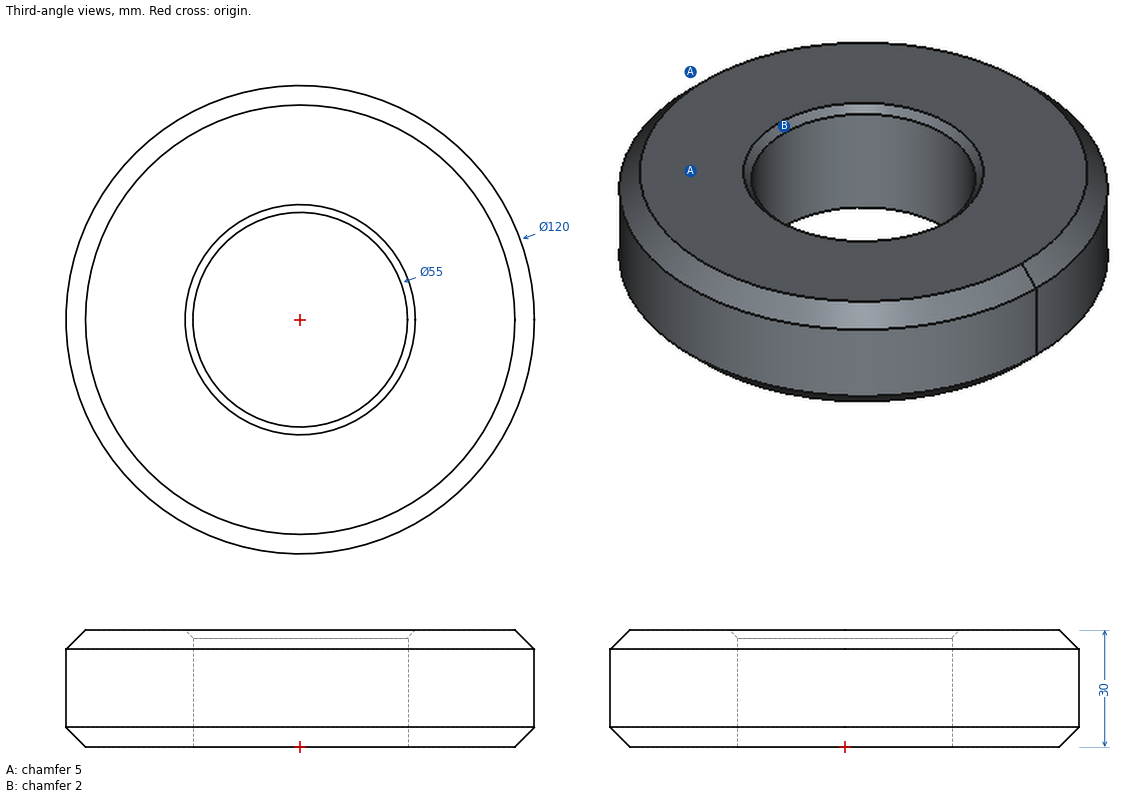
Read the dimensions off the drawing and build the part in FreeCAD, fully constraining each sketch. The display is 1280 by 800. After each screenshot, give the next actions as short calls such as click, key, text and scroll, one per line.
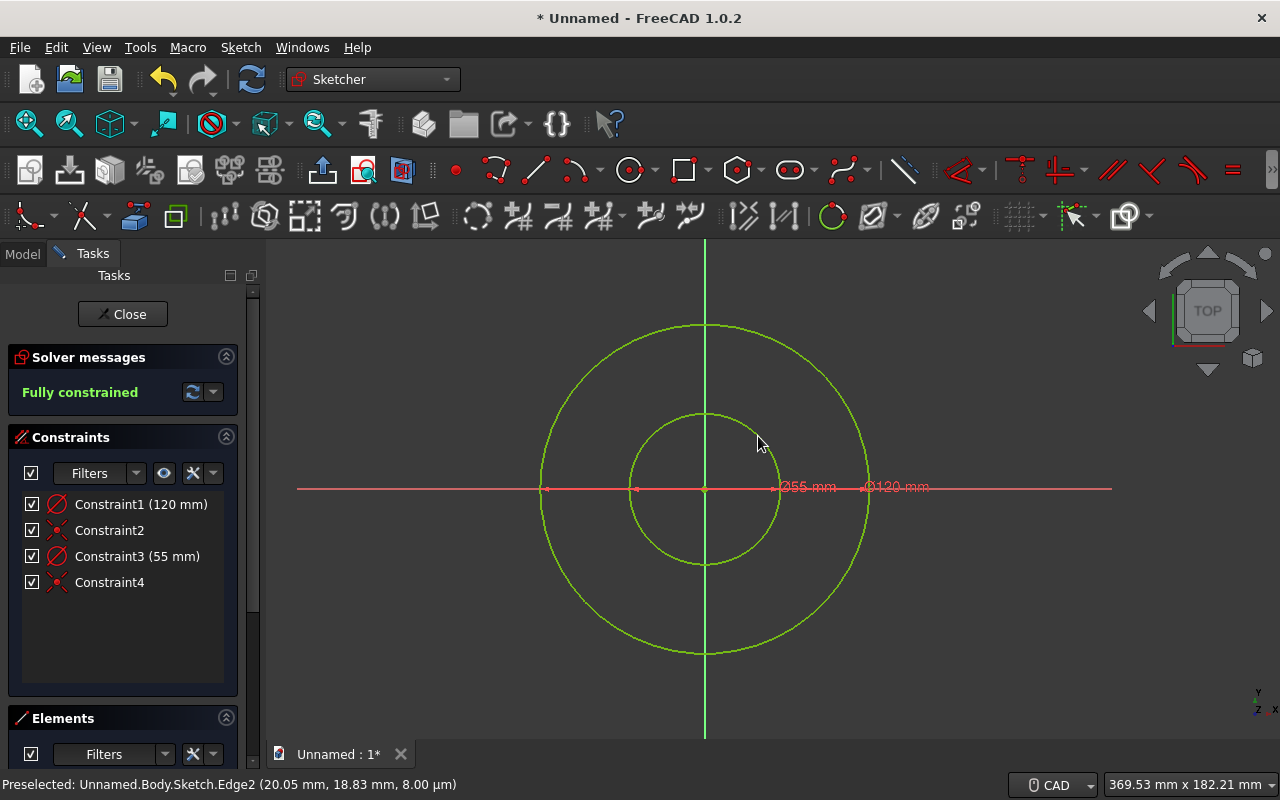
click(123, 314)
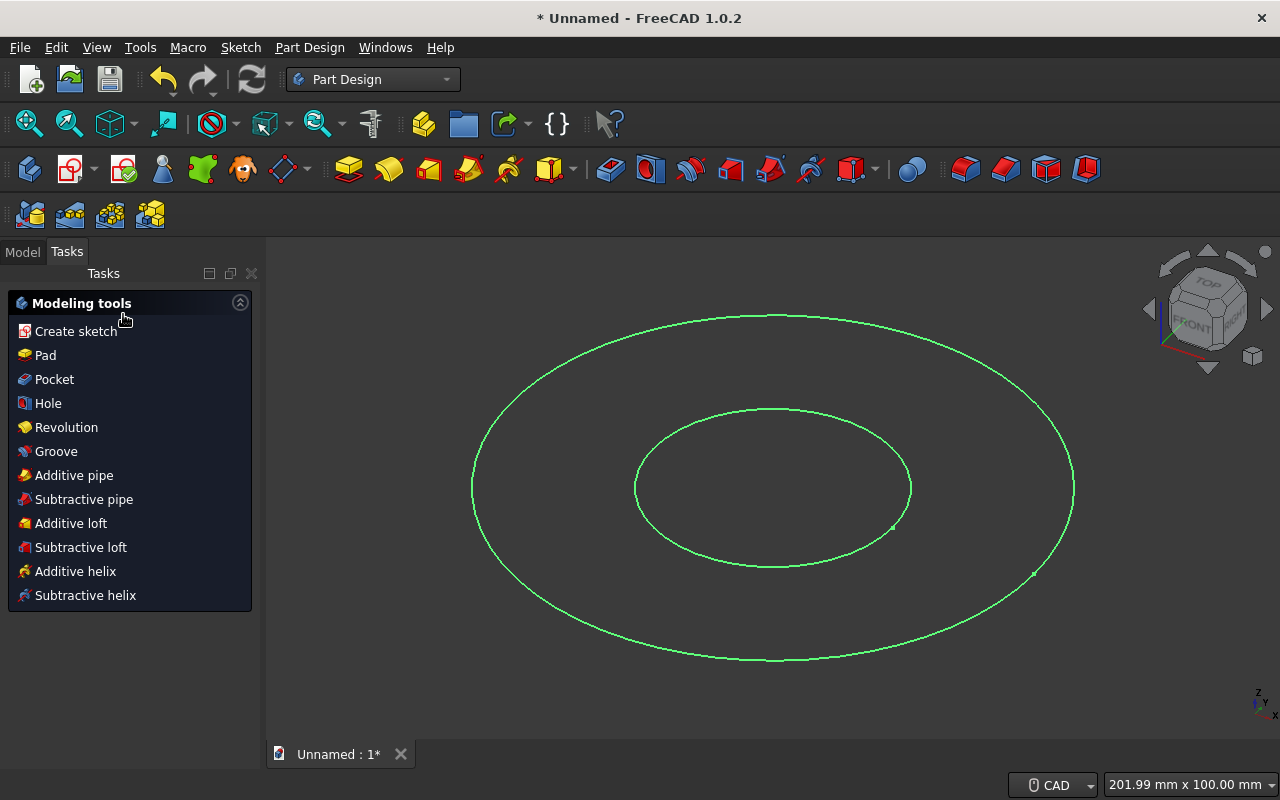
click(350, 170)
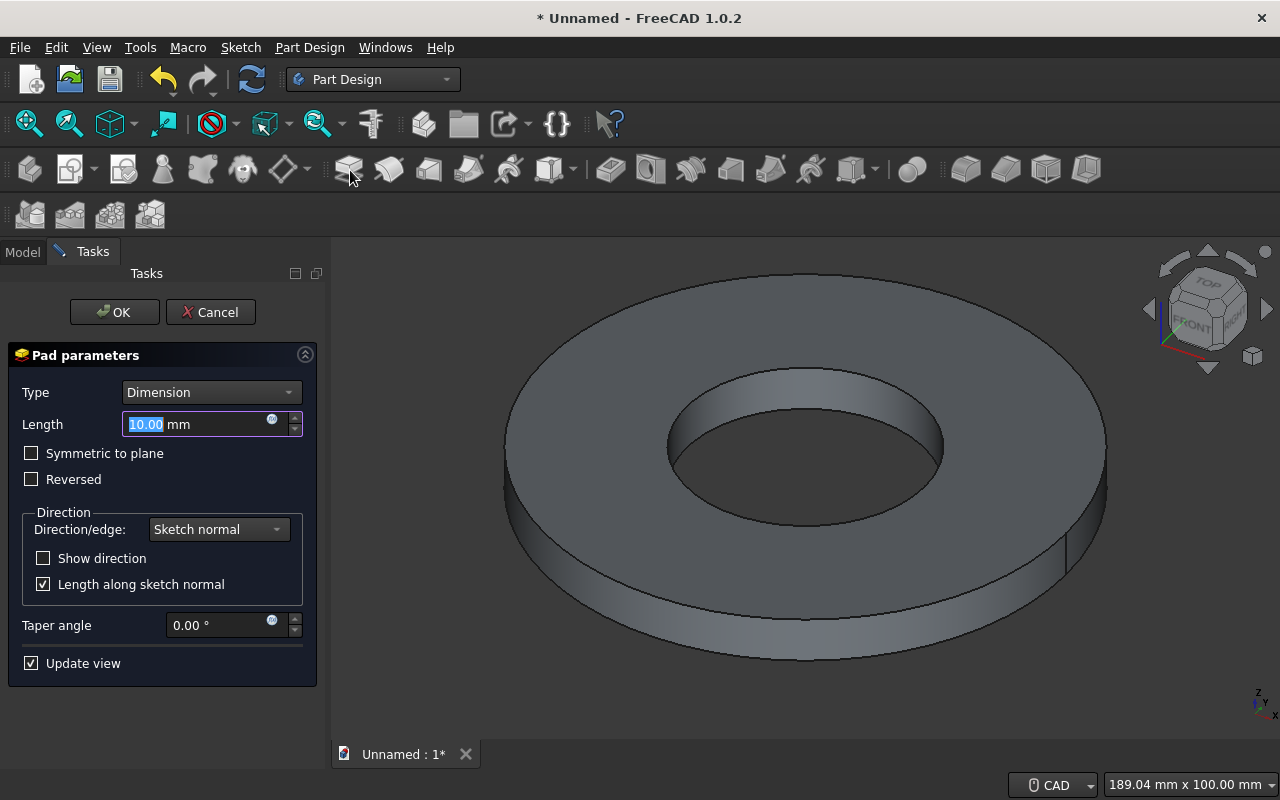
text(30)
key(Tab)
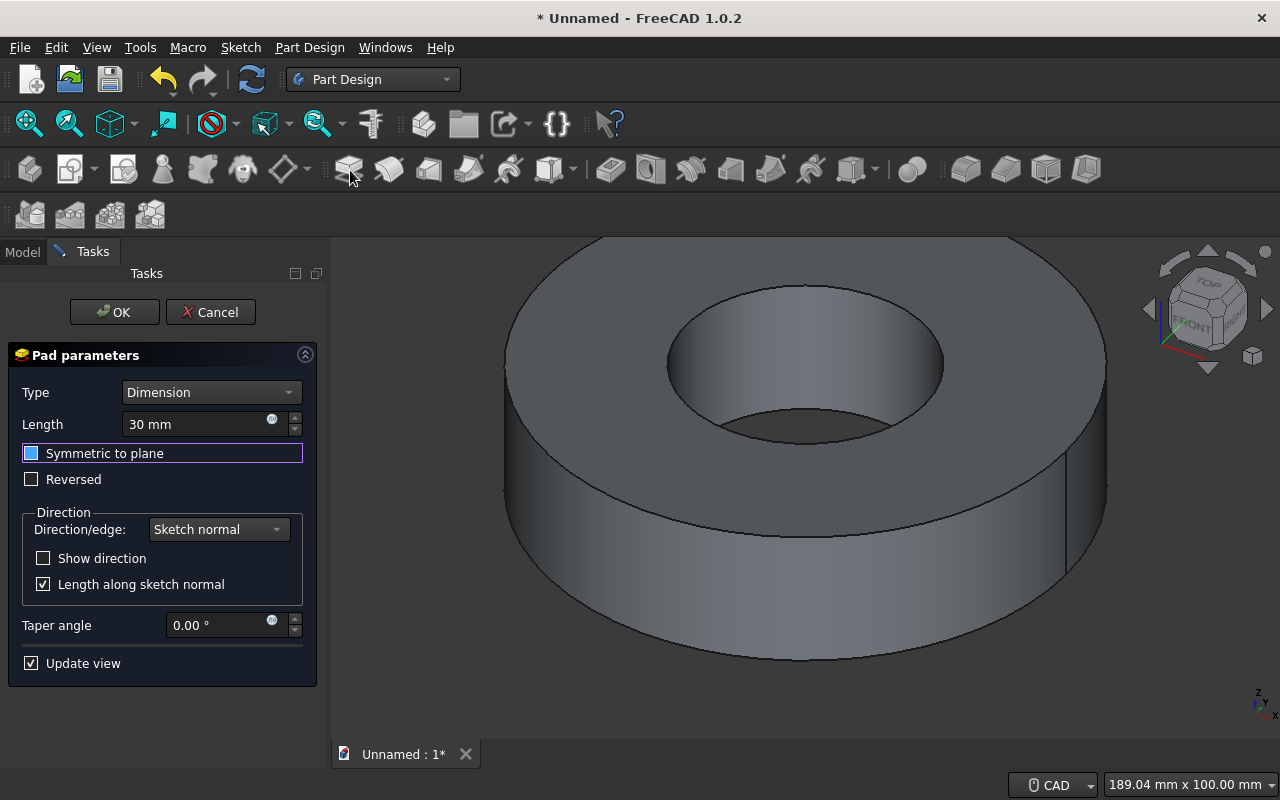
click(115, 312)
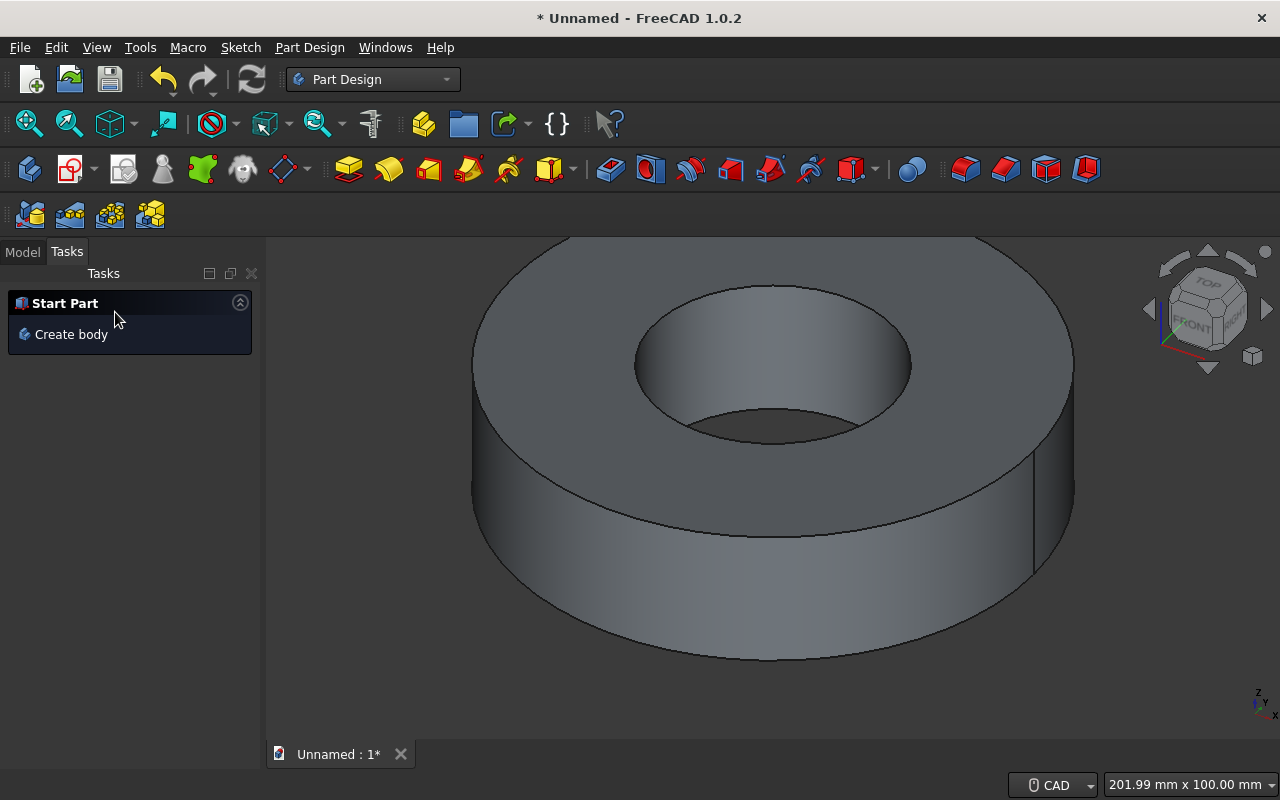
click(30, 124)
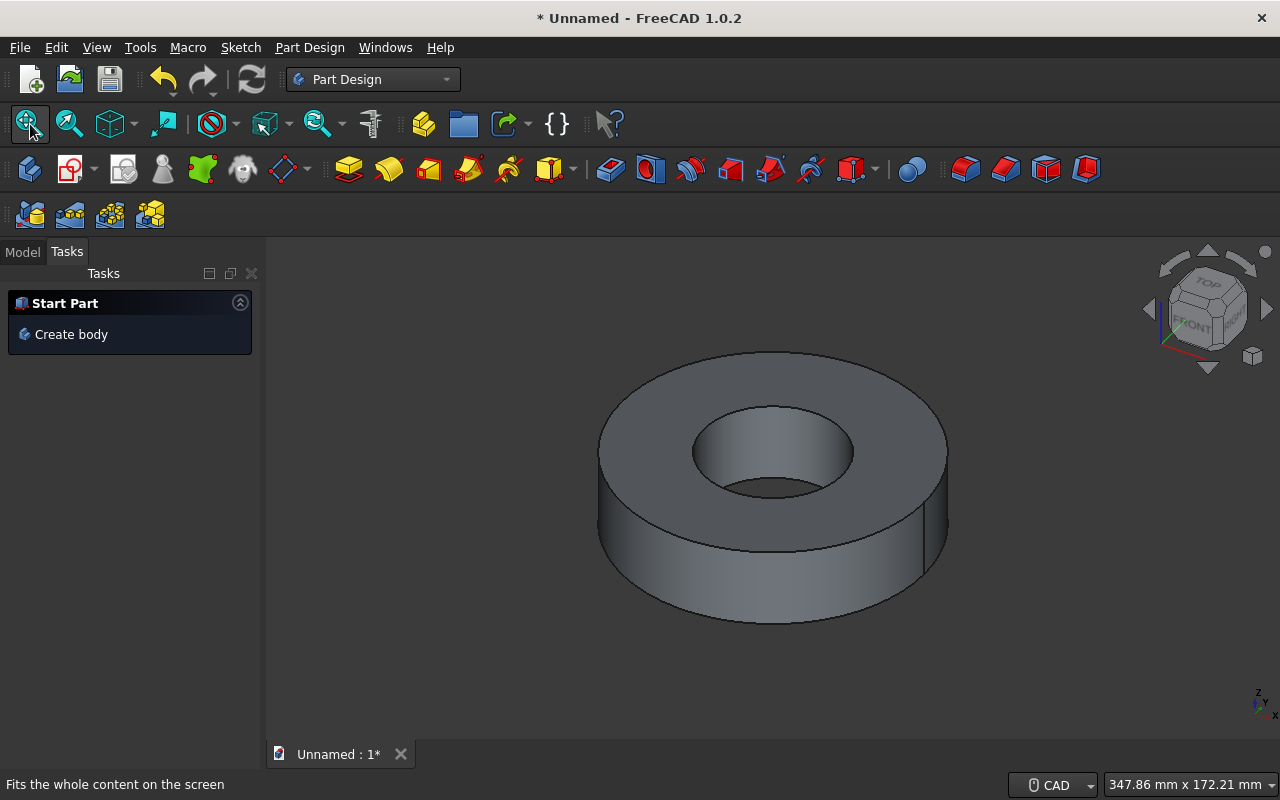
click(599, 462)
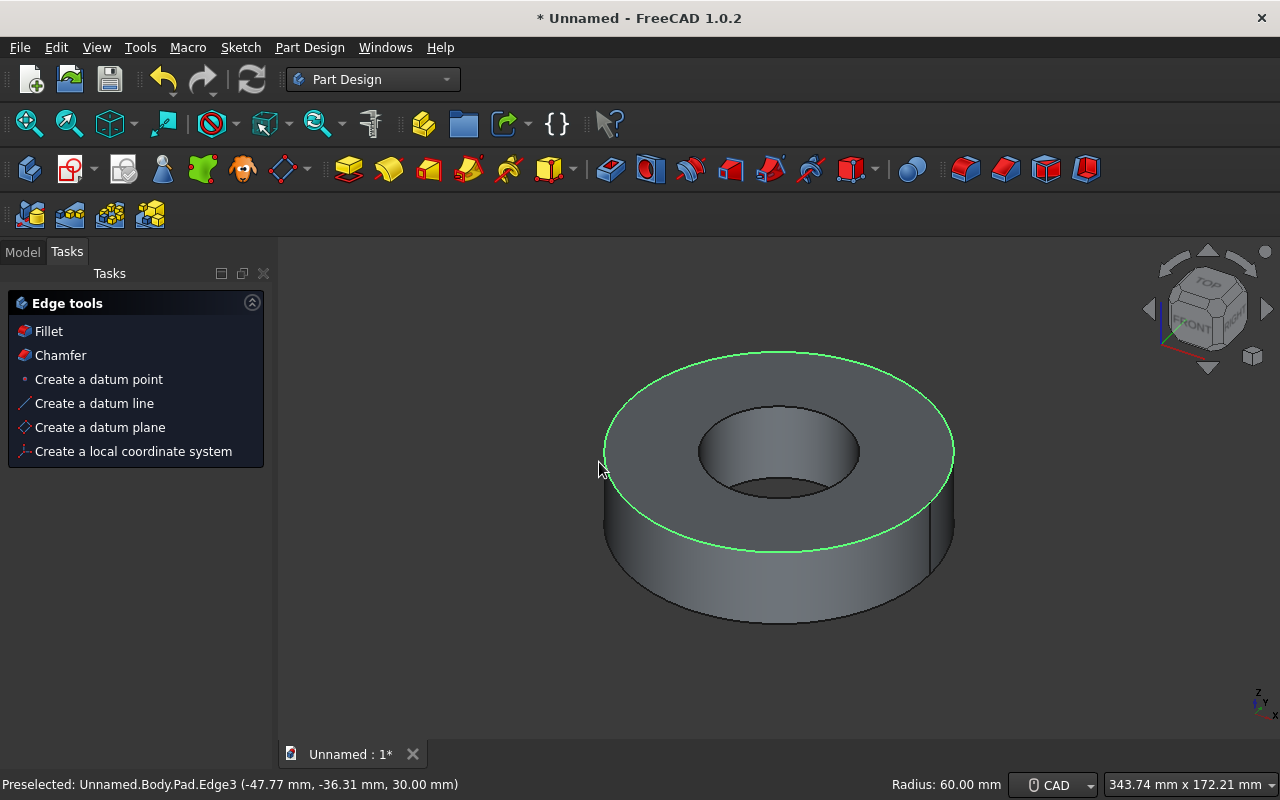
key(0)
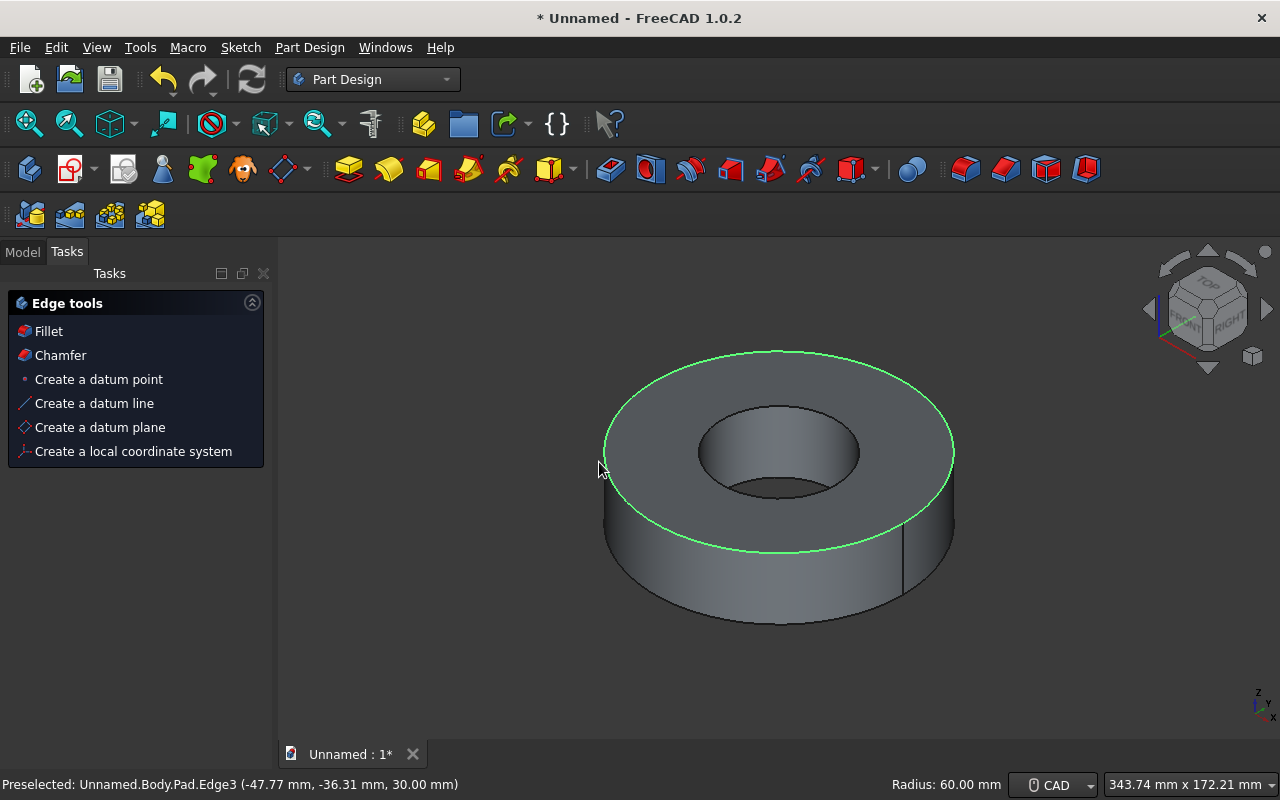
key(2)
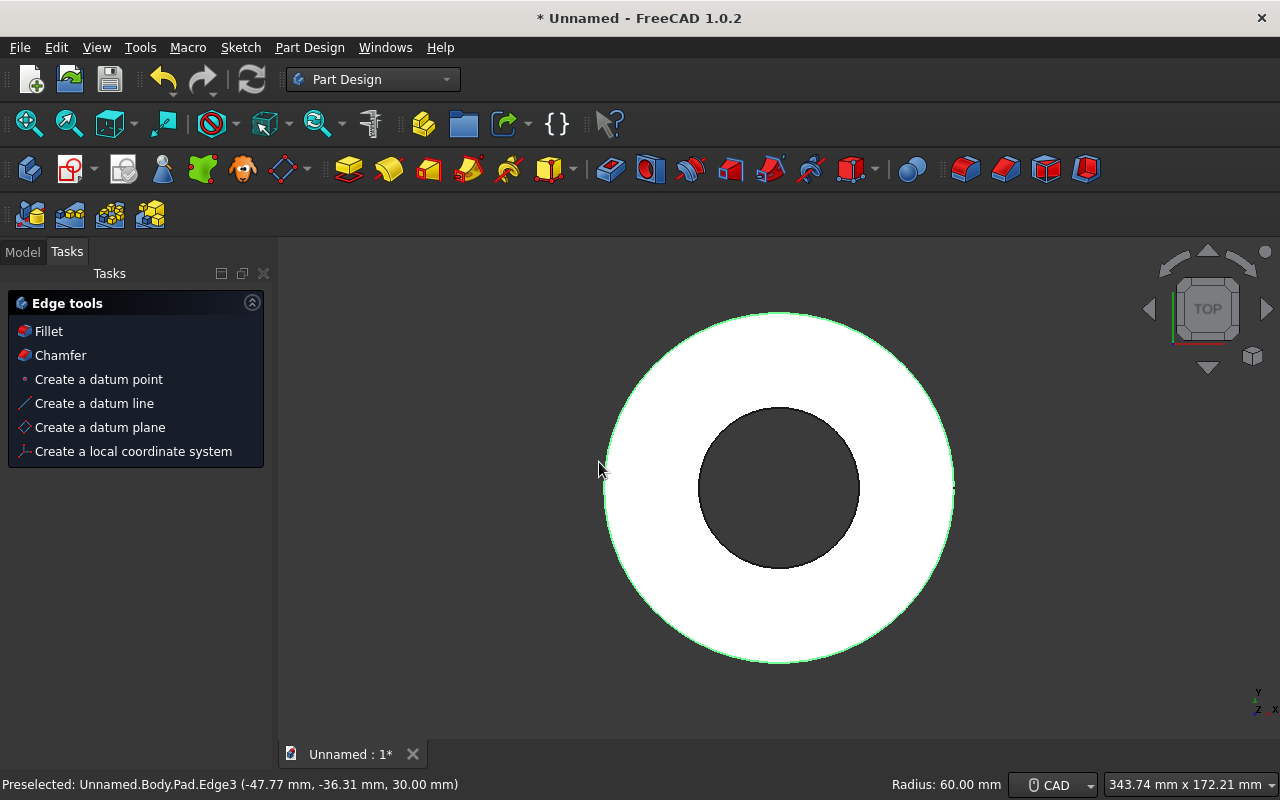
key(1)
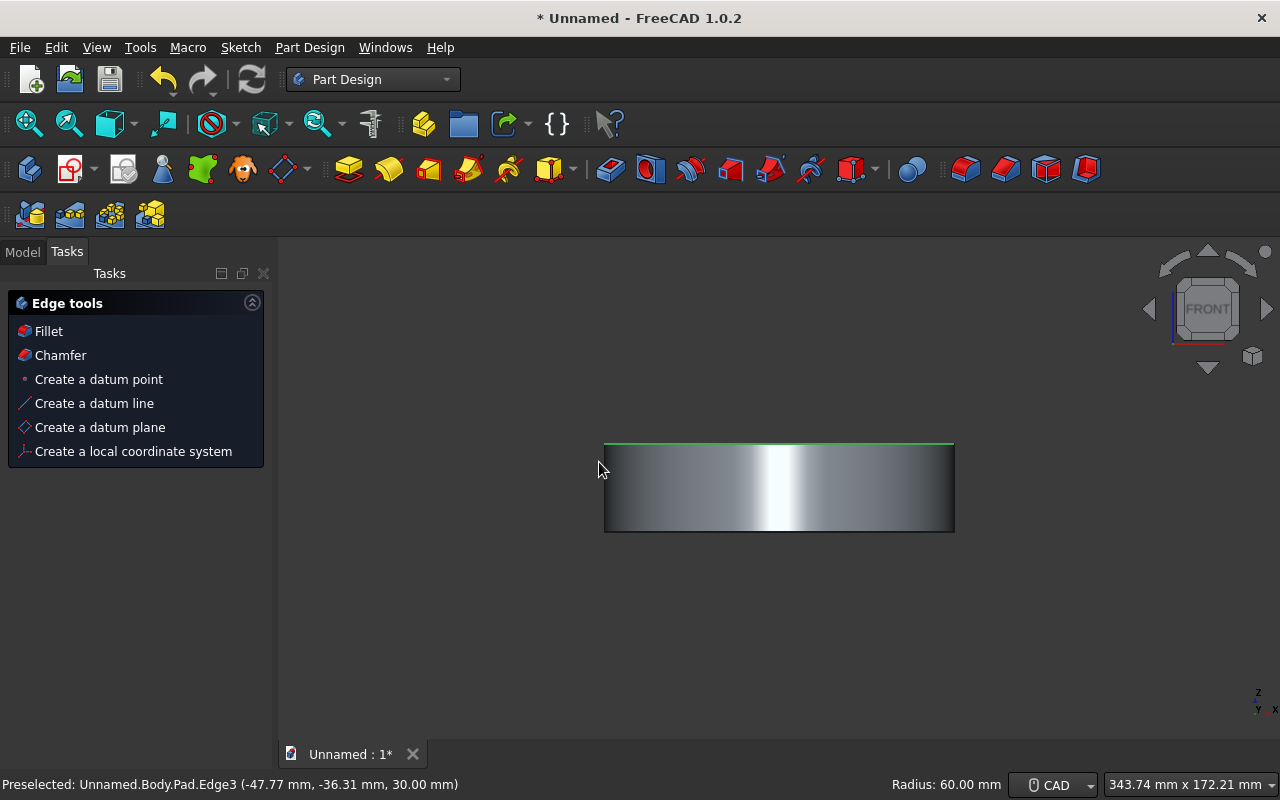
key(v)
key(f)